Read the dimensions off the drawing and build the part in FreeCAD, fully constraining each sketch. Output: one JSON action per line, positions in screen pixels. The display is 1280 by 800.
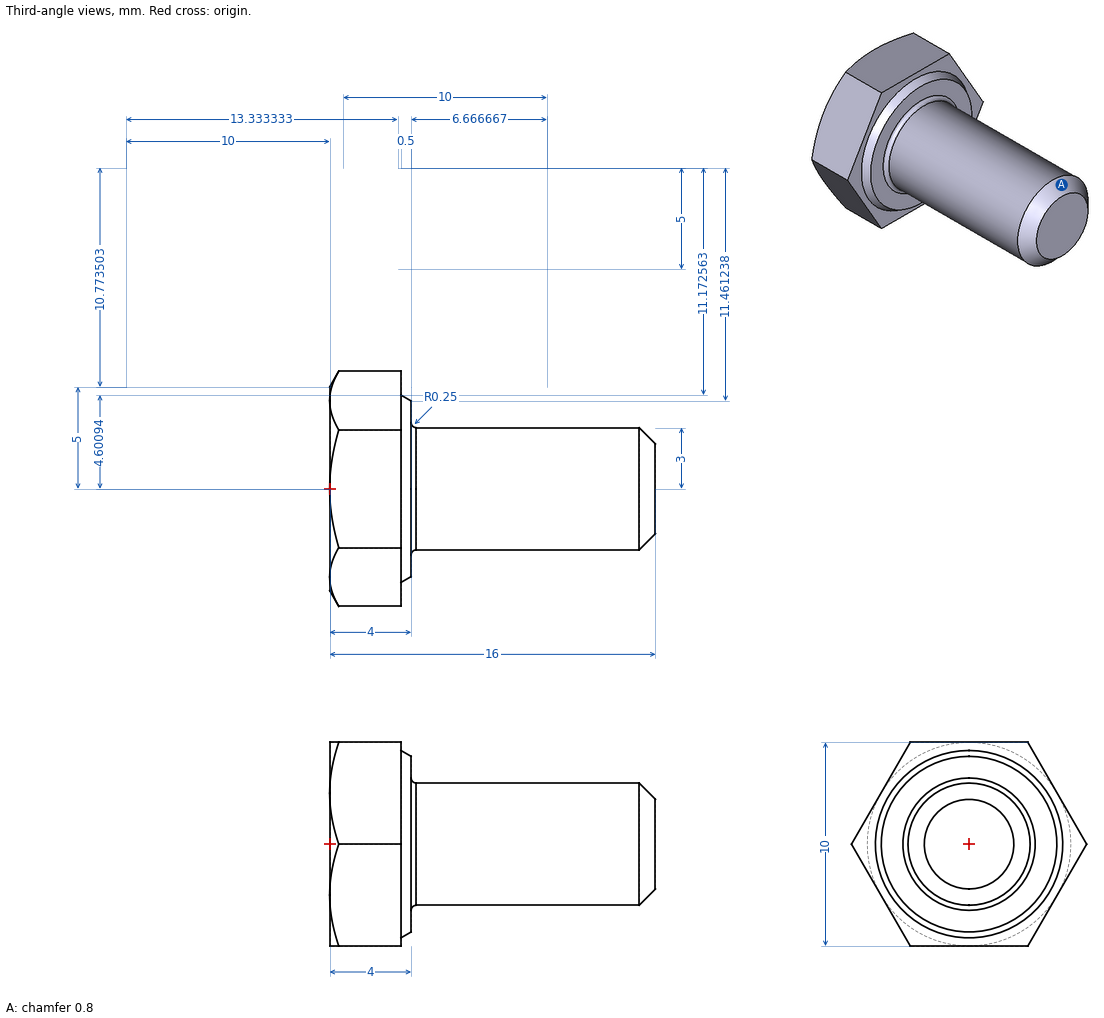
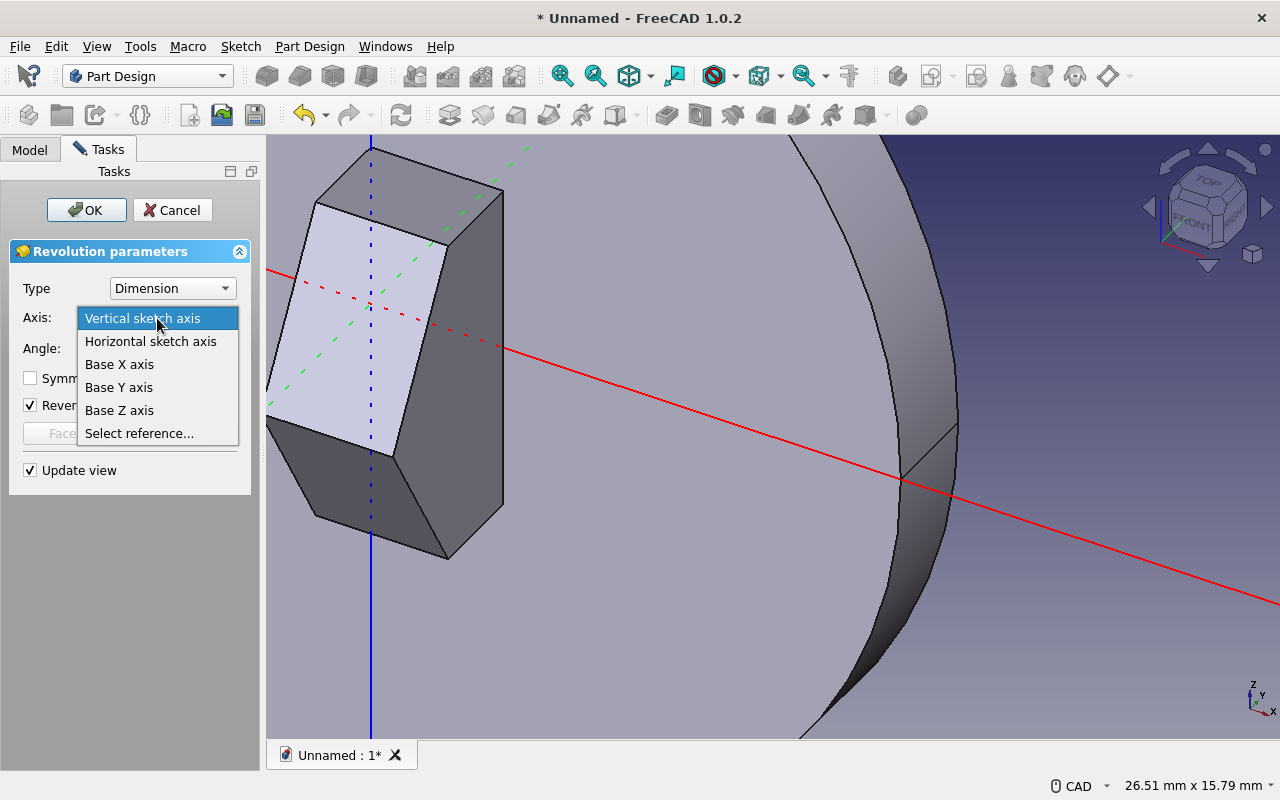
{"action": "left_click", "coordinate": [156, 342]}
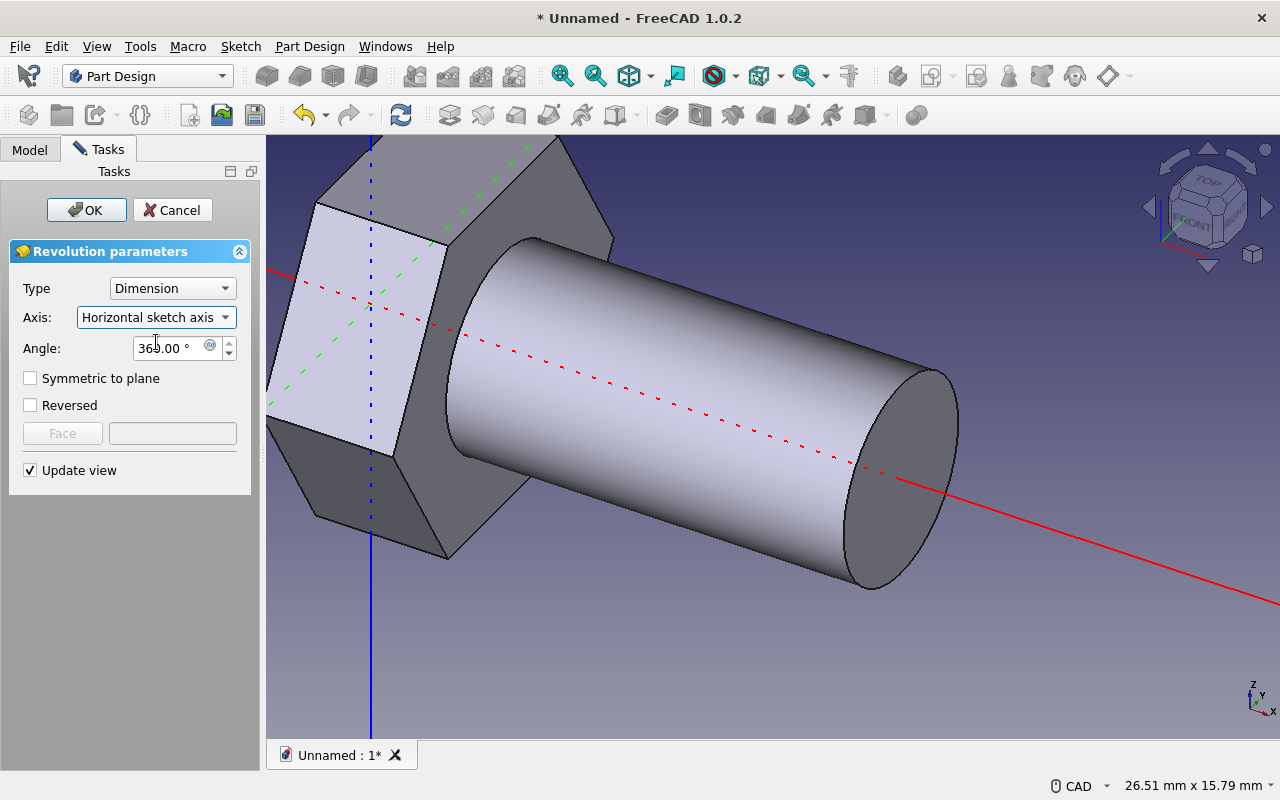
{"action": "left_click", "coordinate": [87, 210]}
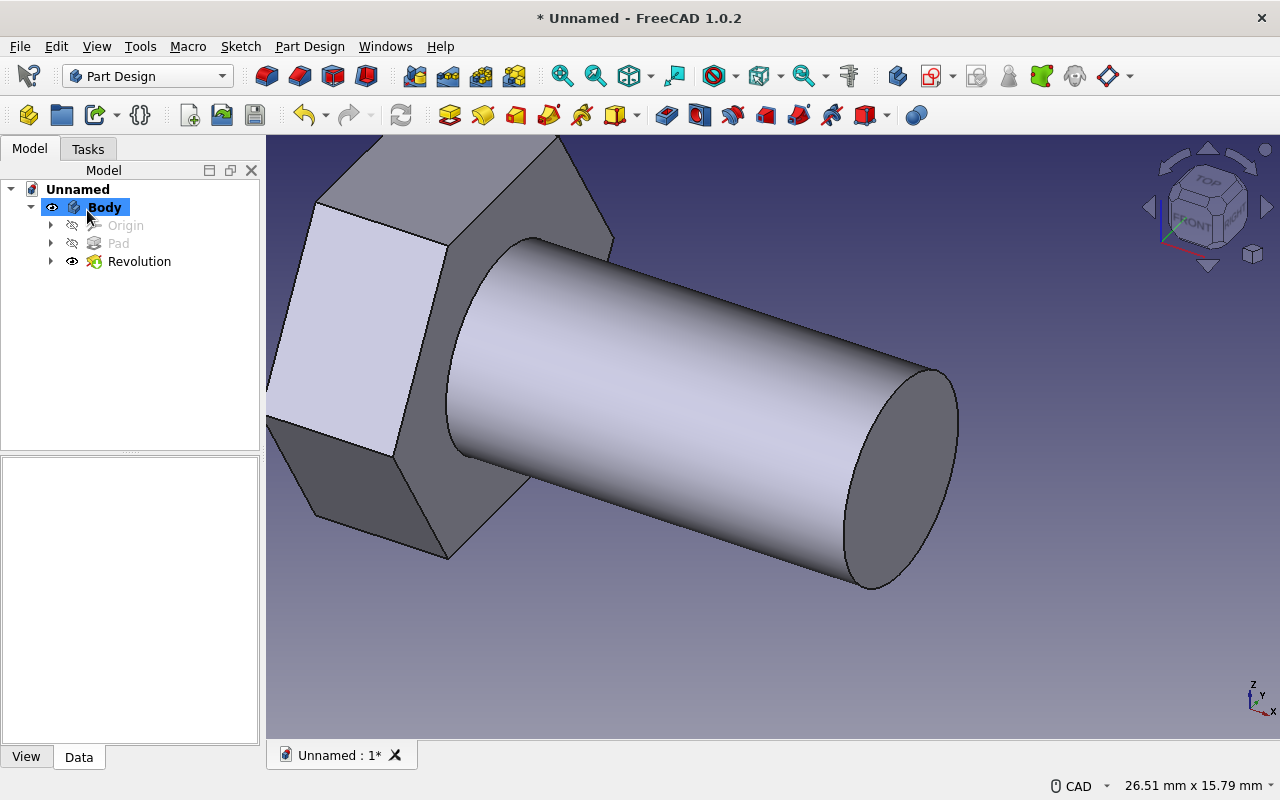
{"action": "left_click", "coordinate": [563, 76]}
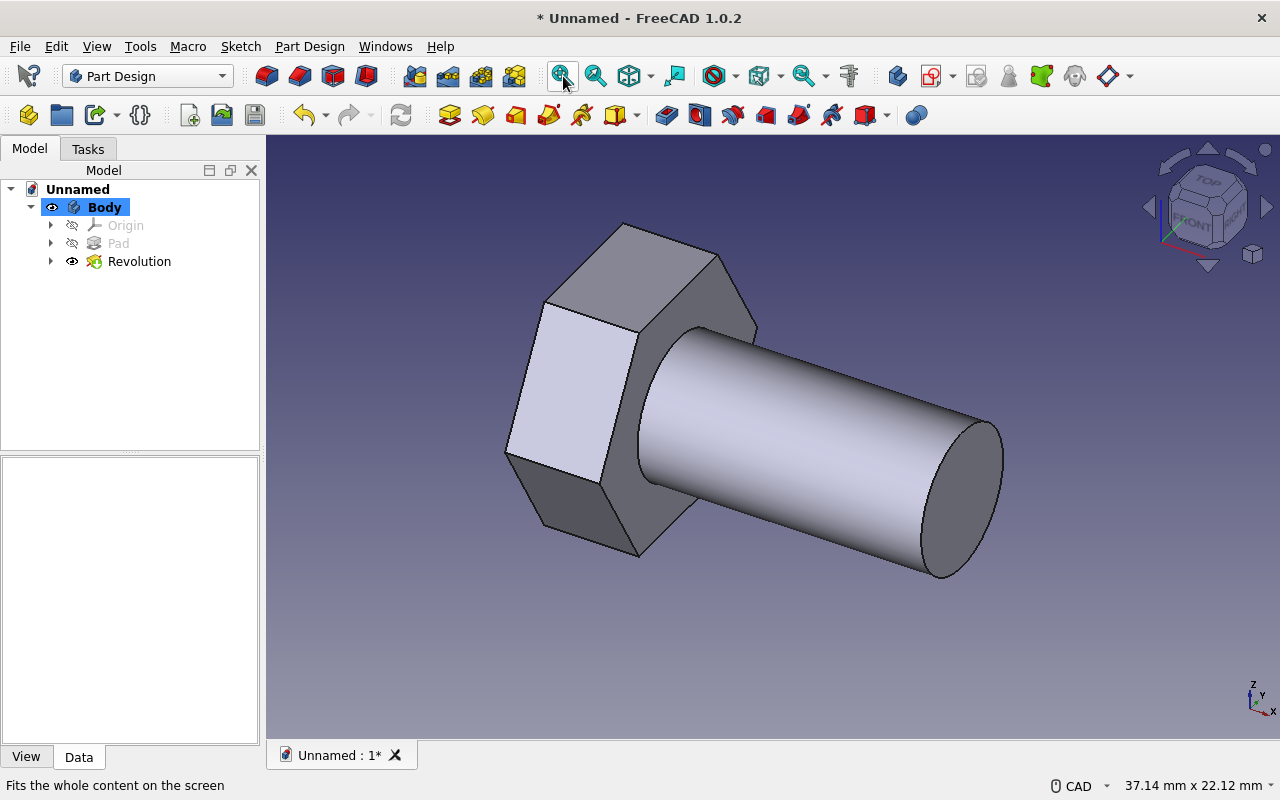
{"action": "left_click", "coordinate": [930, 76]}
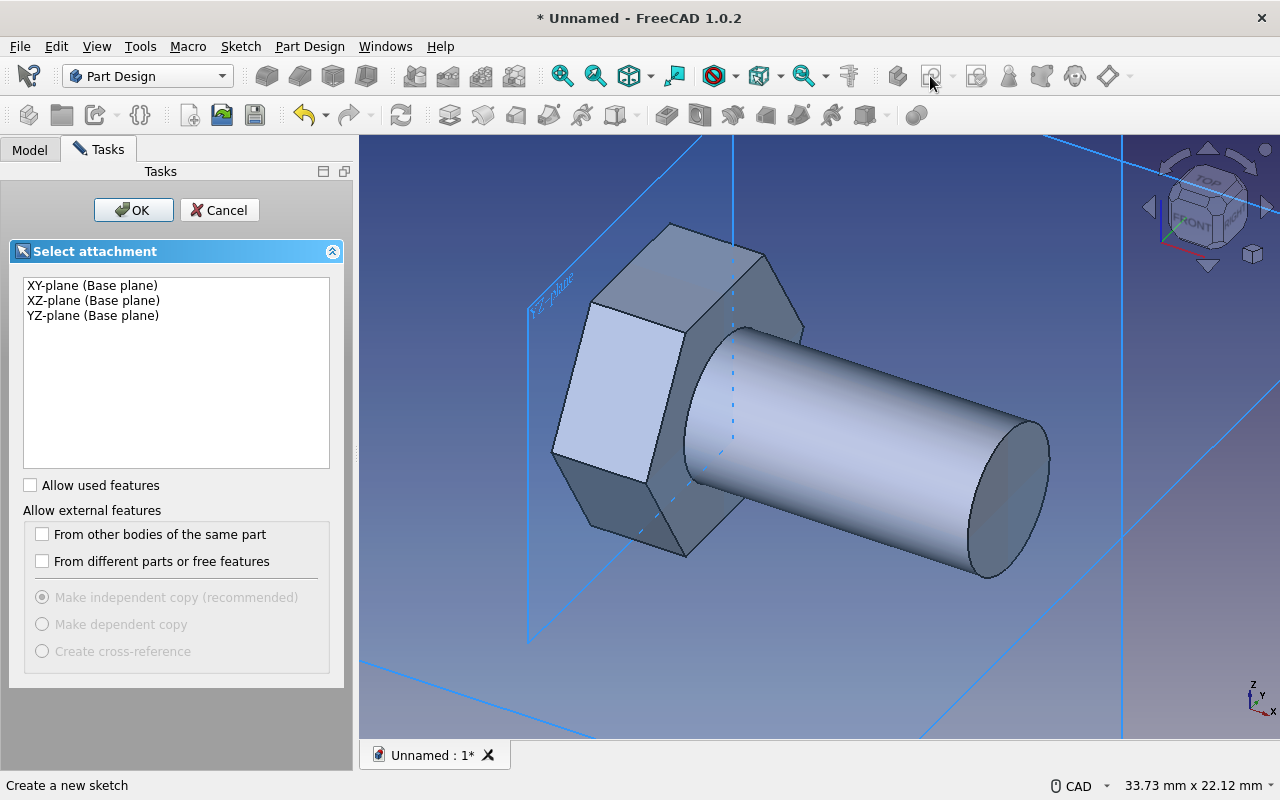
{"action": "left_click", "coordinate": [84, 286]}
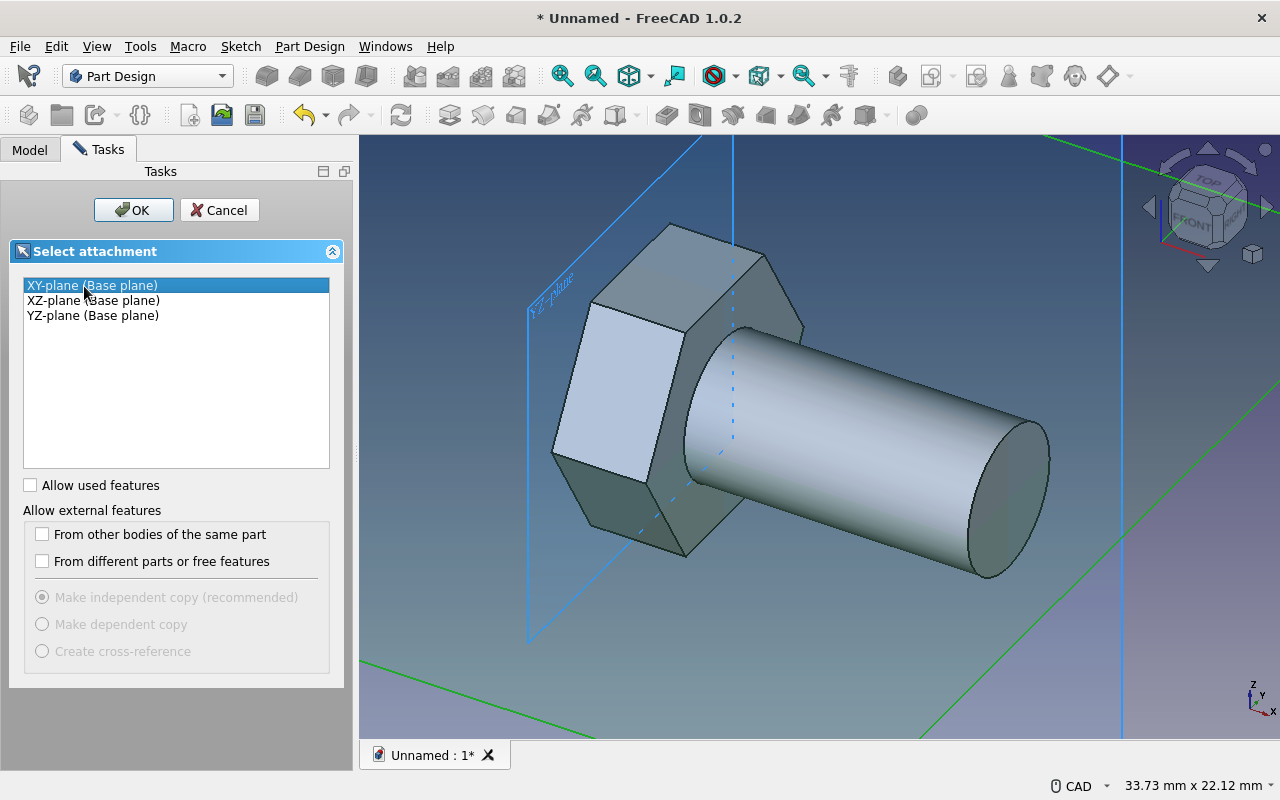
{"action": "left_click", "coordinate": [134, 210]}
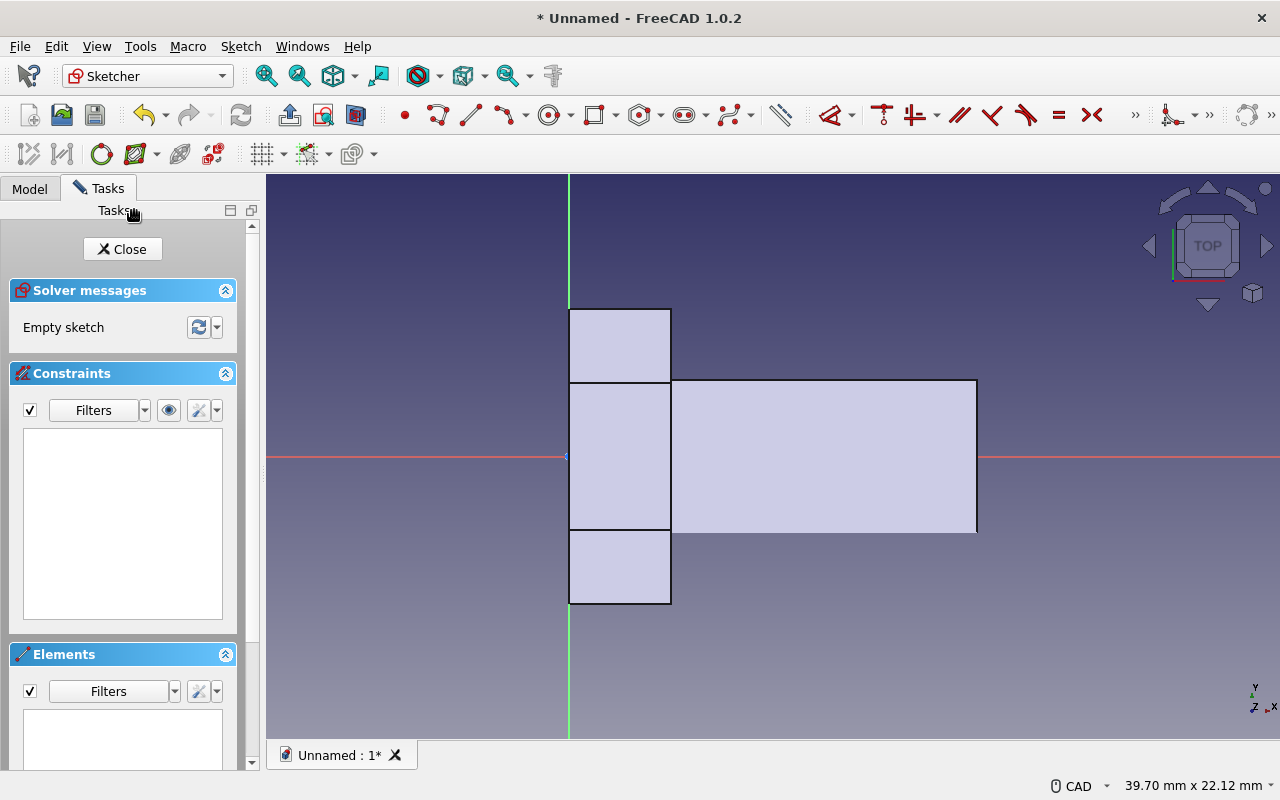
{"action": "left_click", "coordinate": [356, 116]}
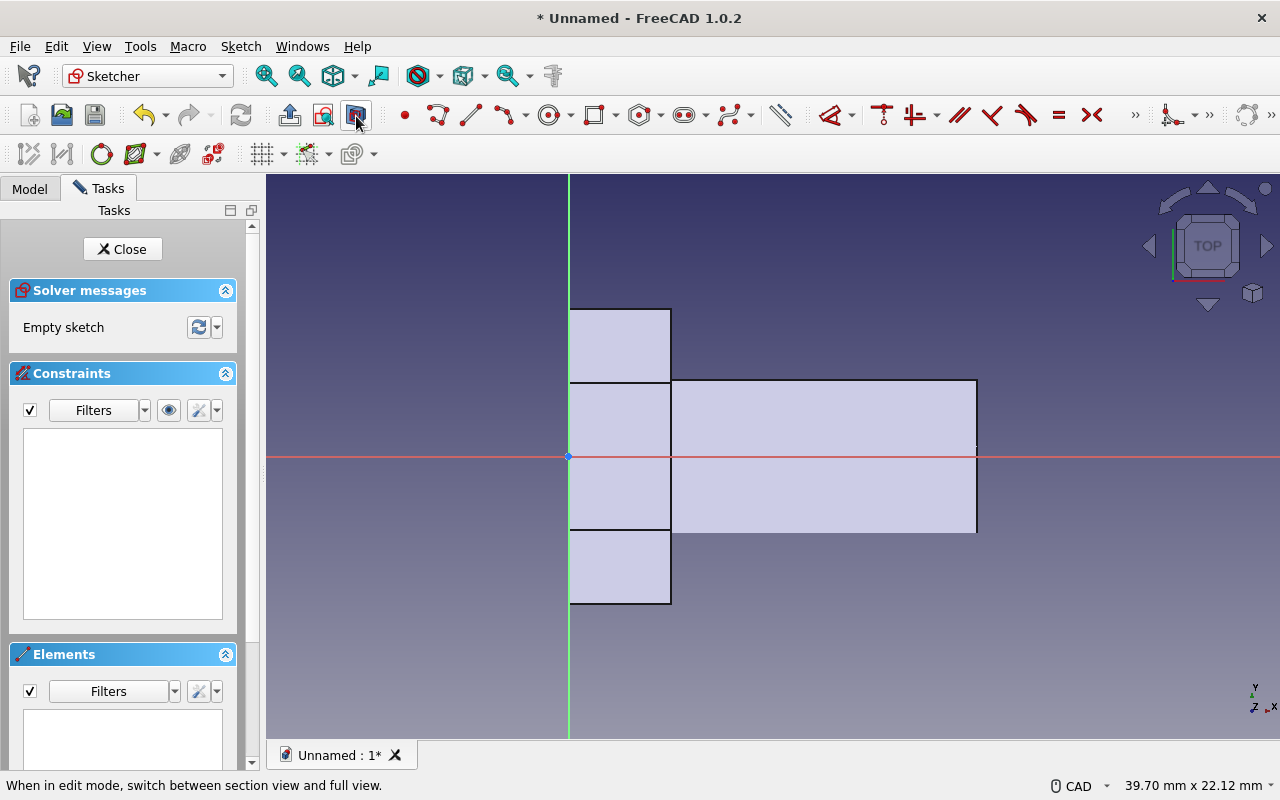
{"action": "scroll", "coordinate": [1115, 711], "scroll_direction": "down", "scroll_amount": 2}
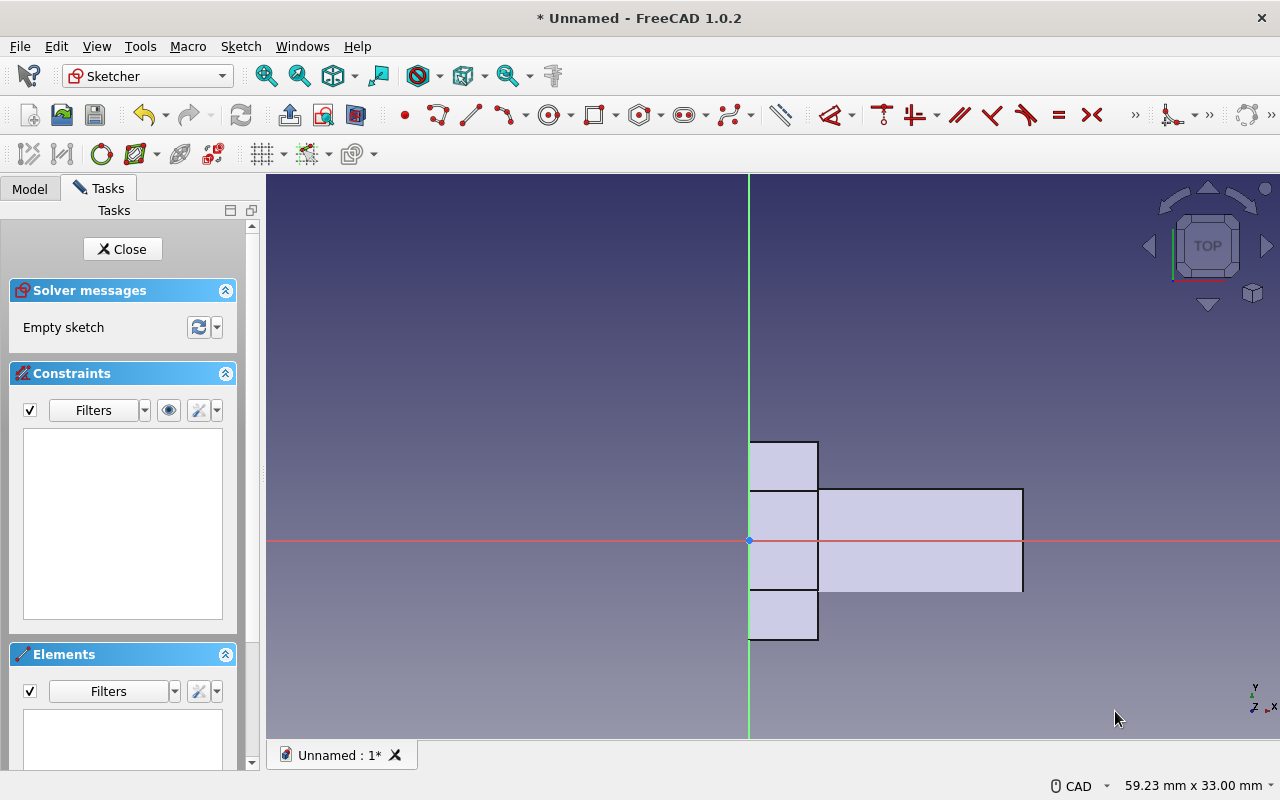
{"action": "left_click", "coordinate": [438, 116]}